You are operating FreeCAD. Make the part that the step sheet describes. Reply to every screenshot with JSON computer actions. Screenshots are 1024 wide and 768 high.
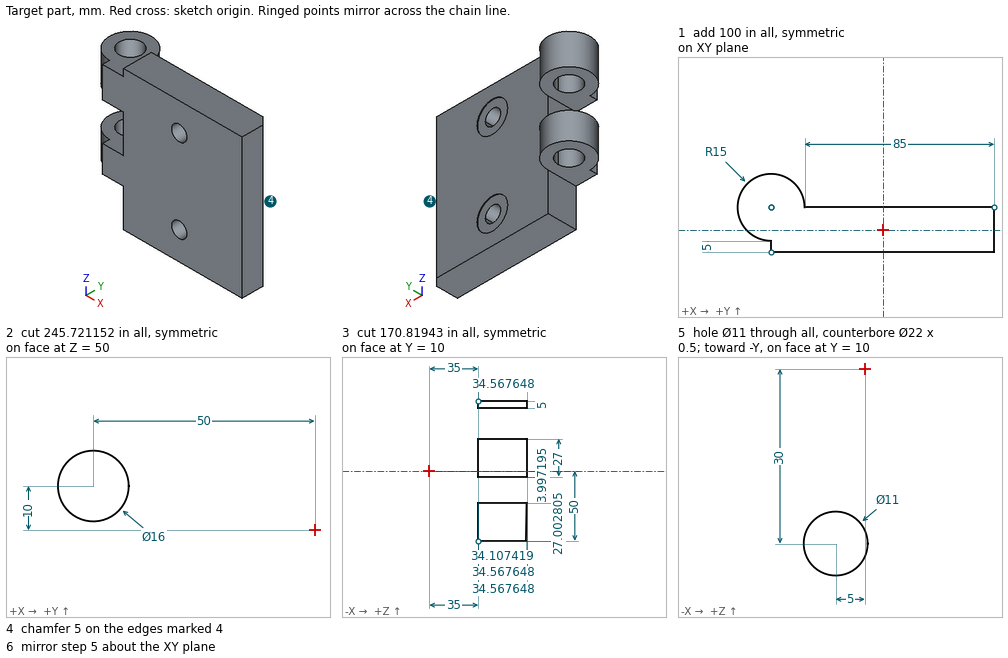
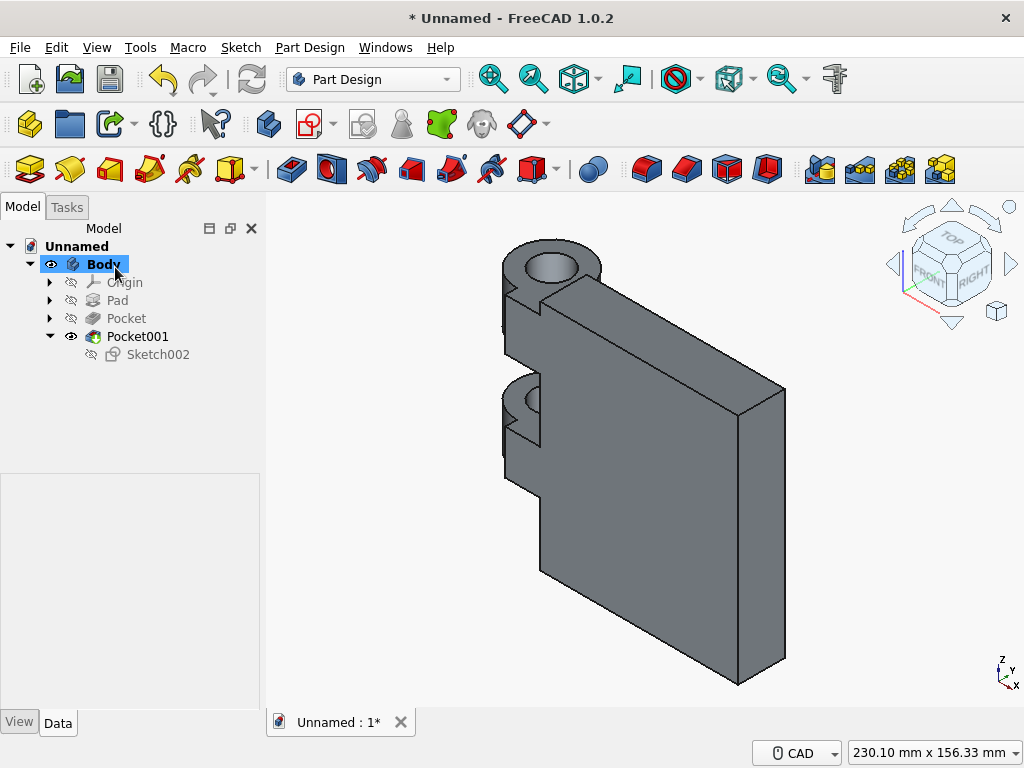
{"action": "key", "text": "2"}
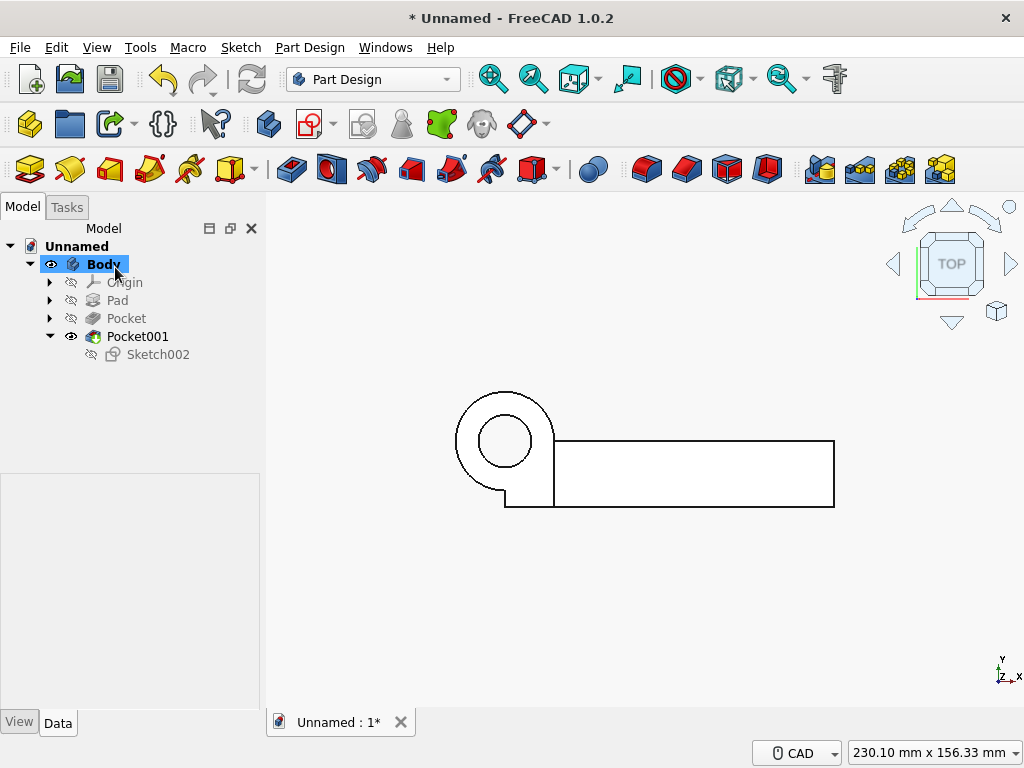
{"action": "key", "text": "1"}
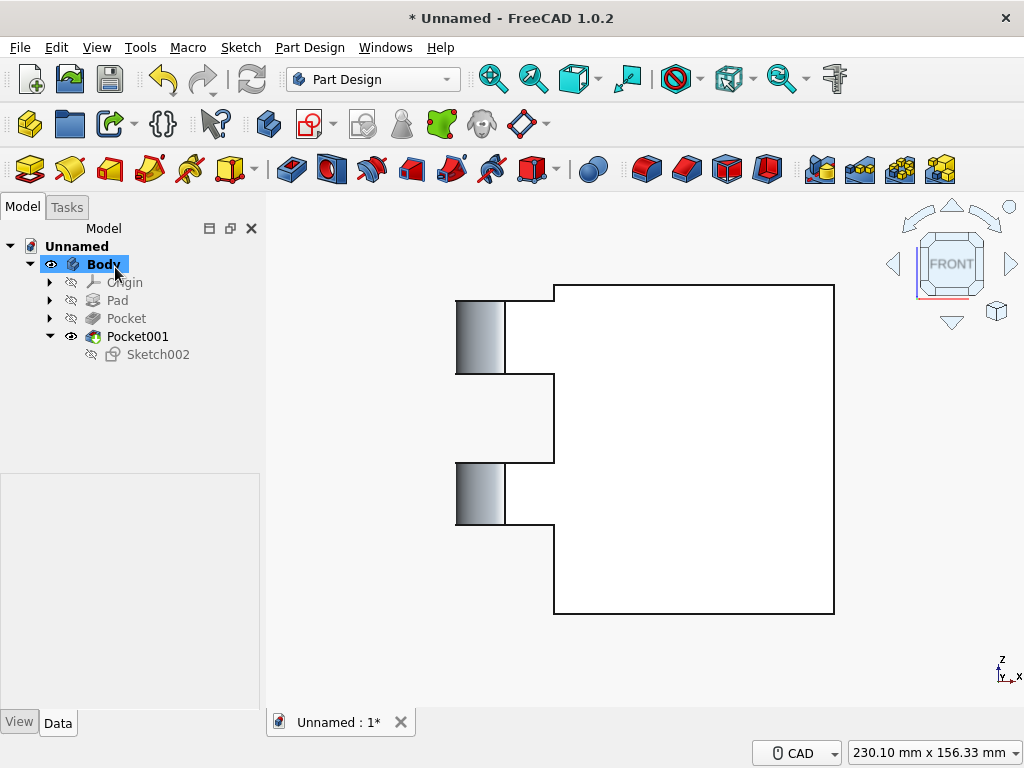
{"action": "key", "text": "3"}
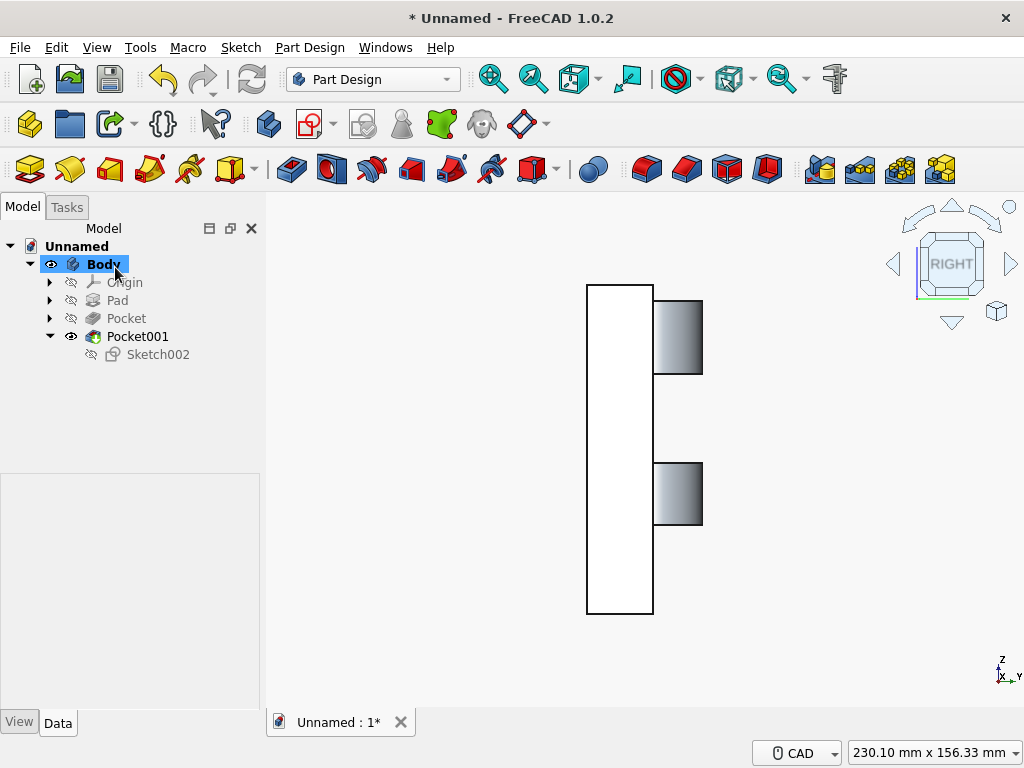
{"action": "left_click", "coordinate": [653, 448]}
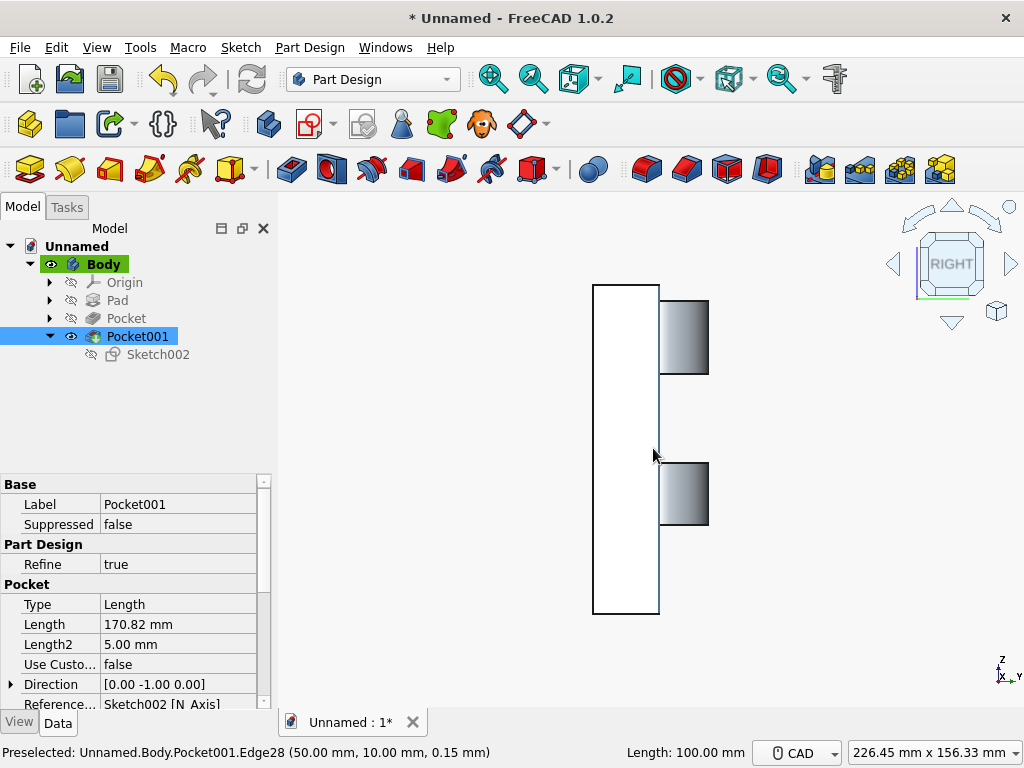
{"action": "left_click", "coordinate": [688, 170]}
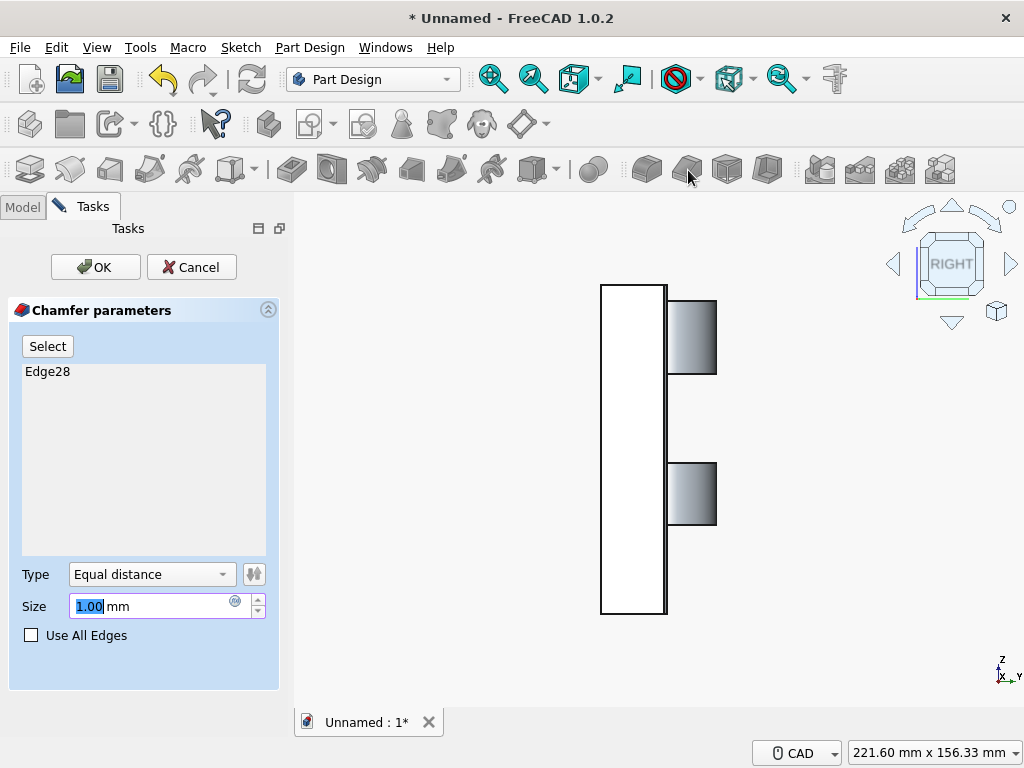
{"action": "type", "text": "5"}
{"action": "key", "text": "Tab"}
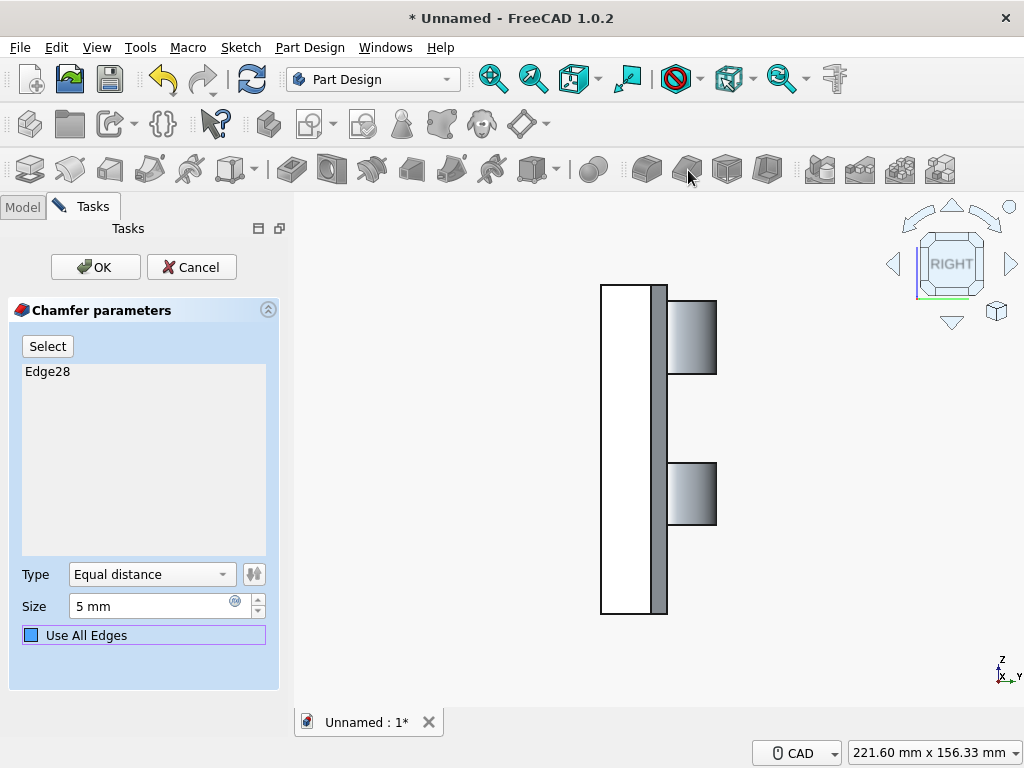
{"action": "left_click", "coordinate": [96, 267]}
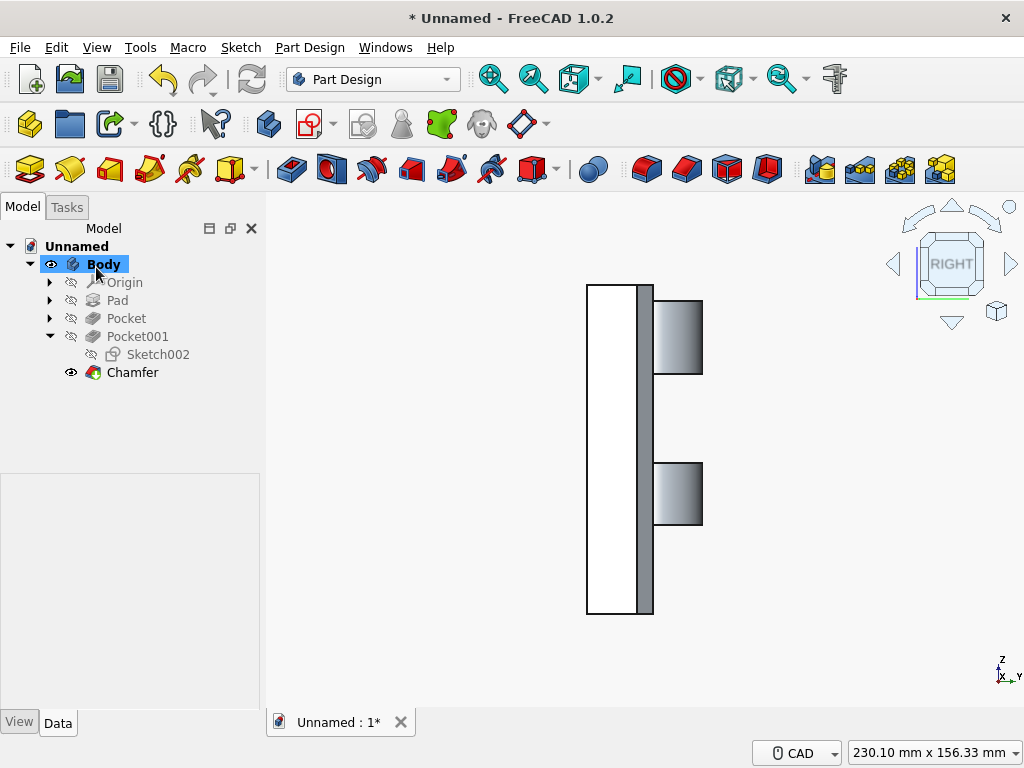
{"action": "key", "text": "4"}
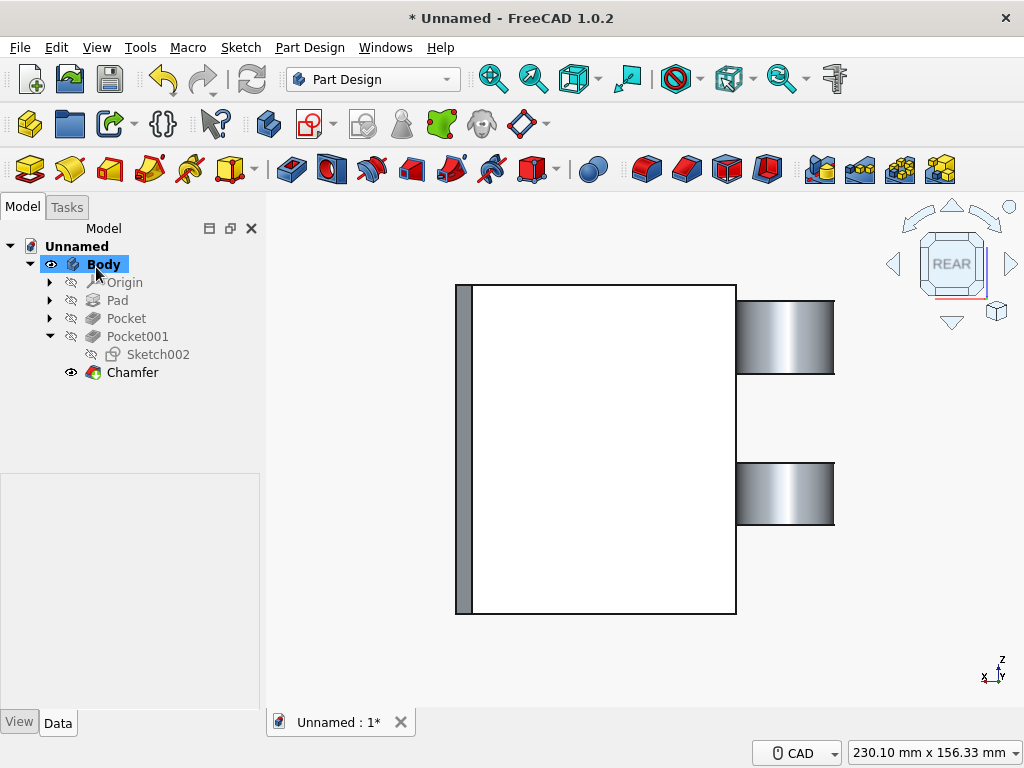
{"action": "left_click", "coordinate": [604, 448]}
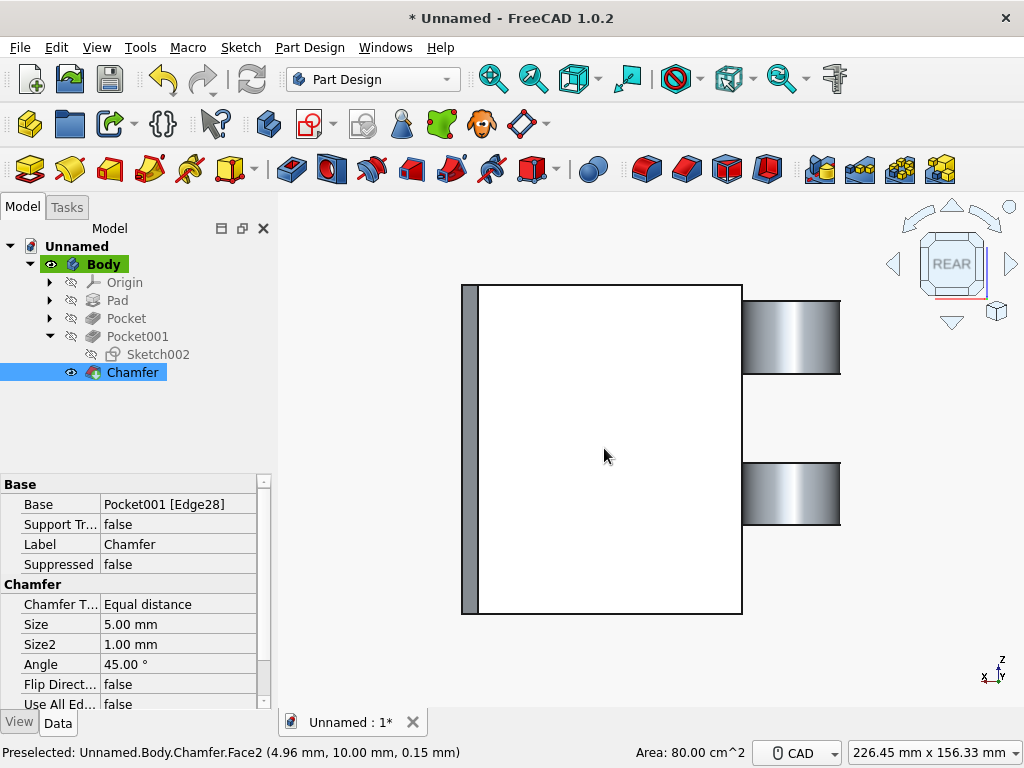
{"action": "left_click", "coordinate": [310, 124]}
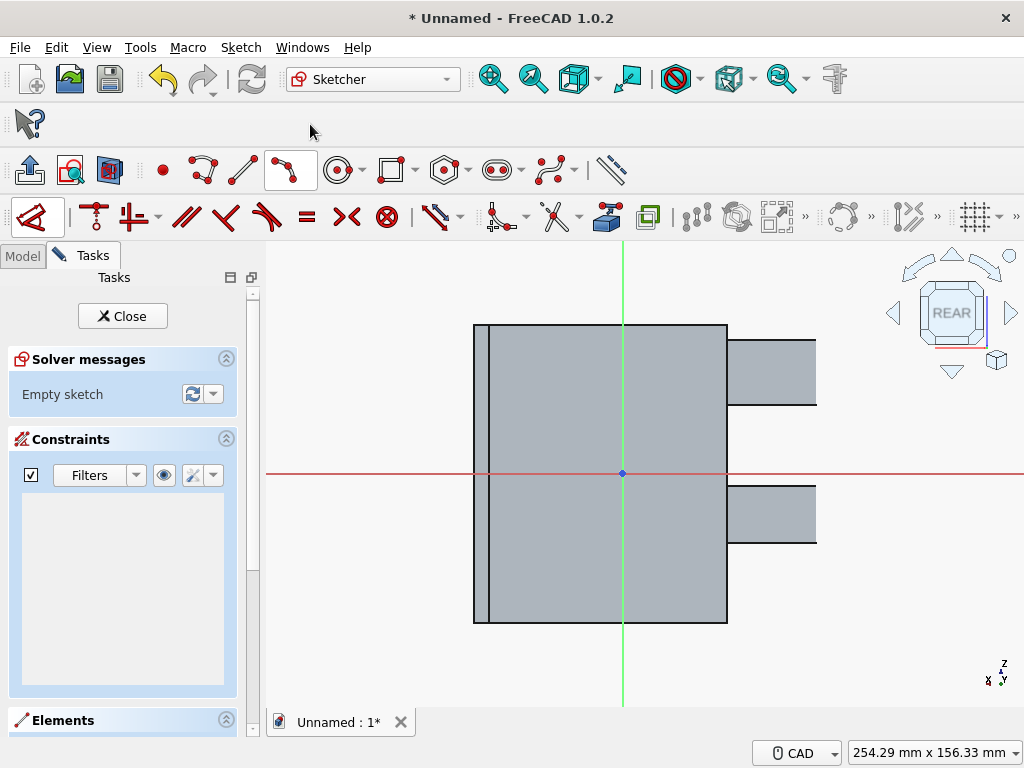
{"action": "left_click", "coordinate": [110, 170]}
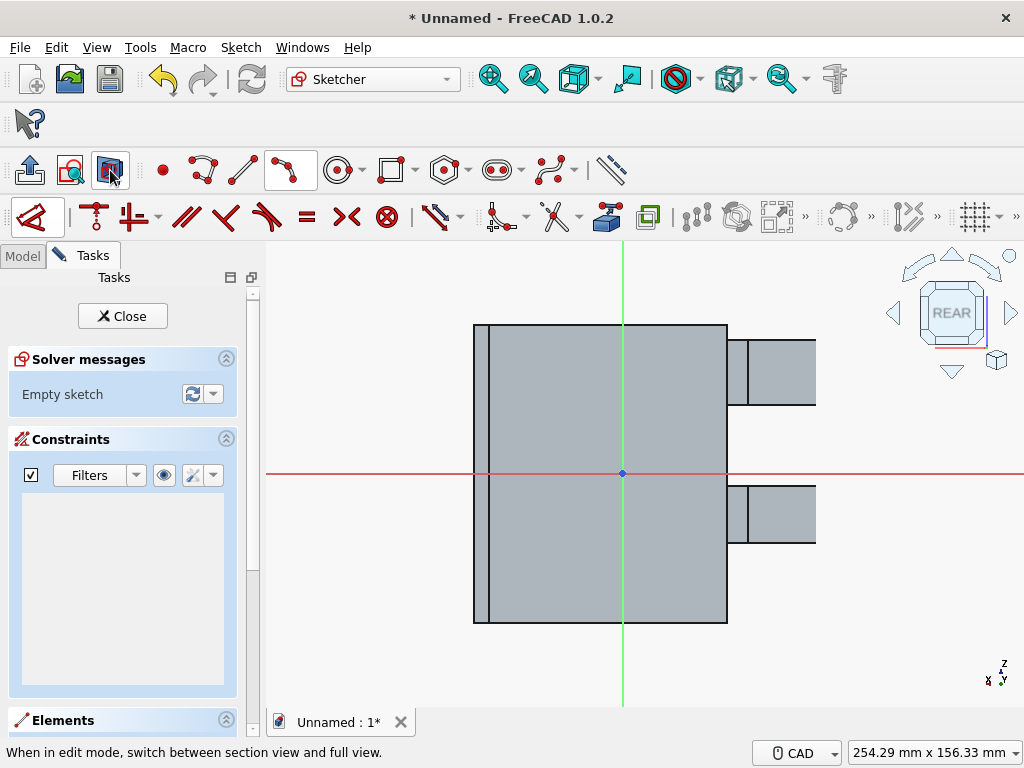
{"action": "scroll", "coordinate": [612, 575], "scroll_direction": "up", "scroll_amount": 11}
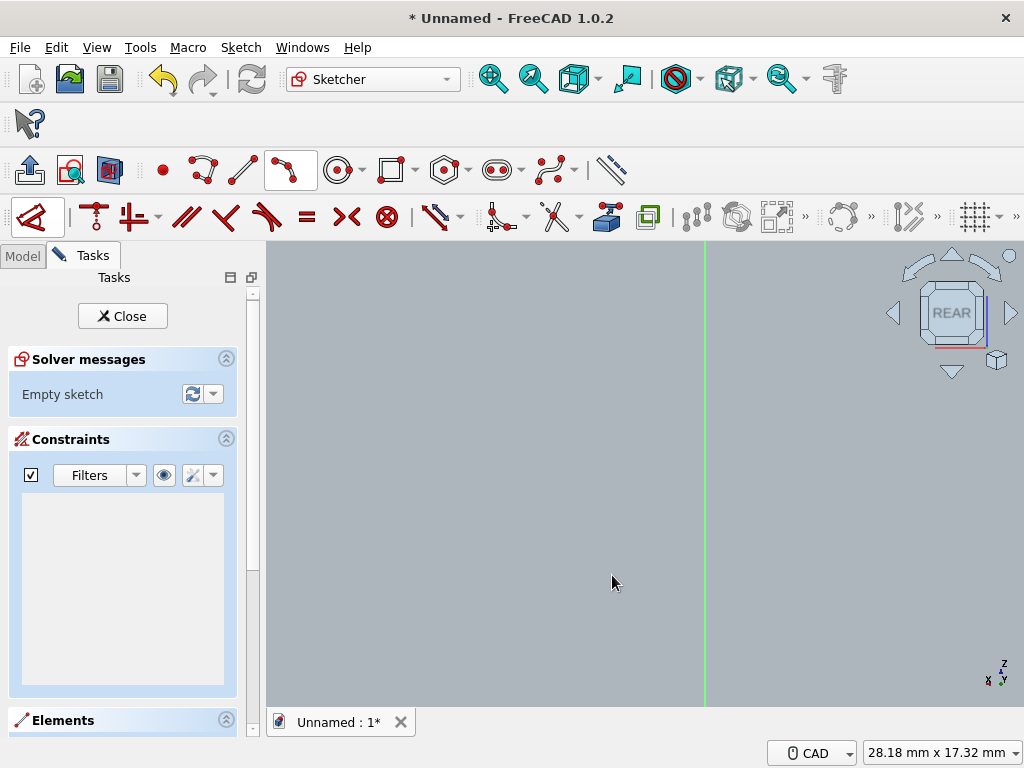
{"action": "left_click", "coordinate": [338, 170]}